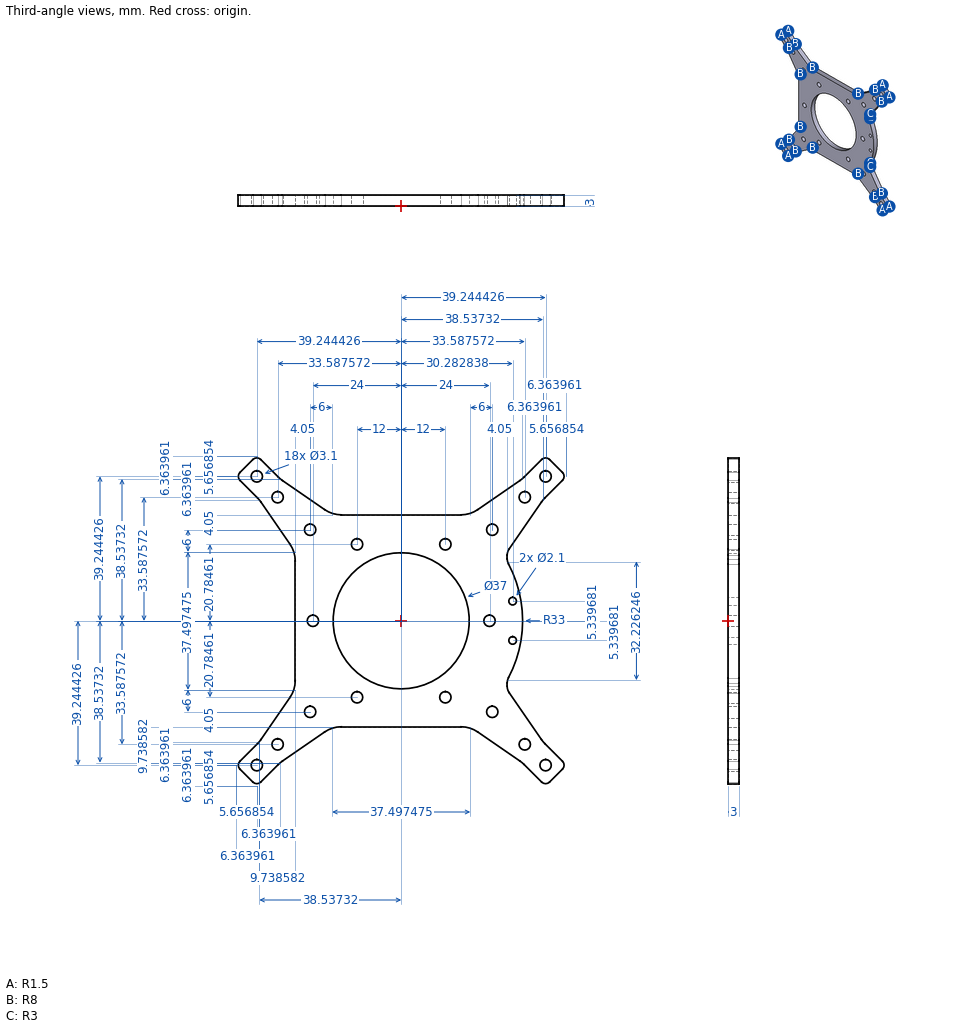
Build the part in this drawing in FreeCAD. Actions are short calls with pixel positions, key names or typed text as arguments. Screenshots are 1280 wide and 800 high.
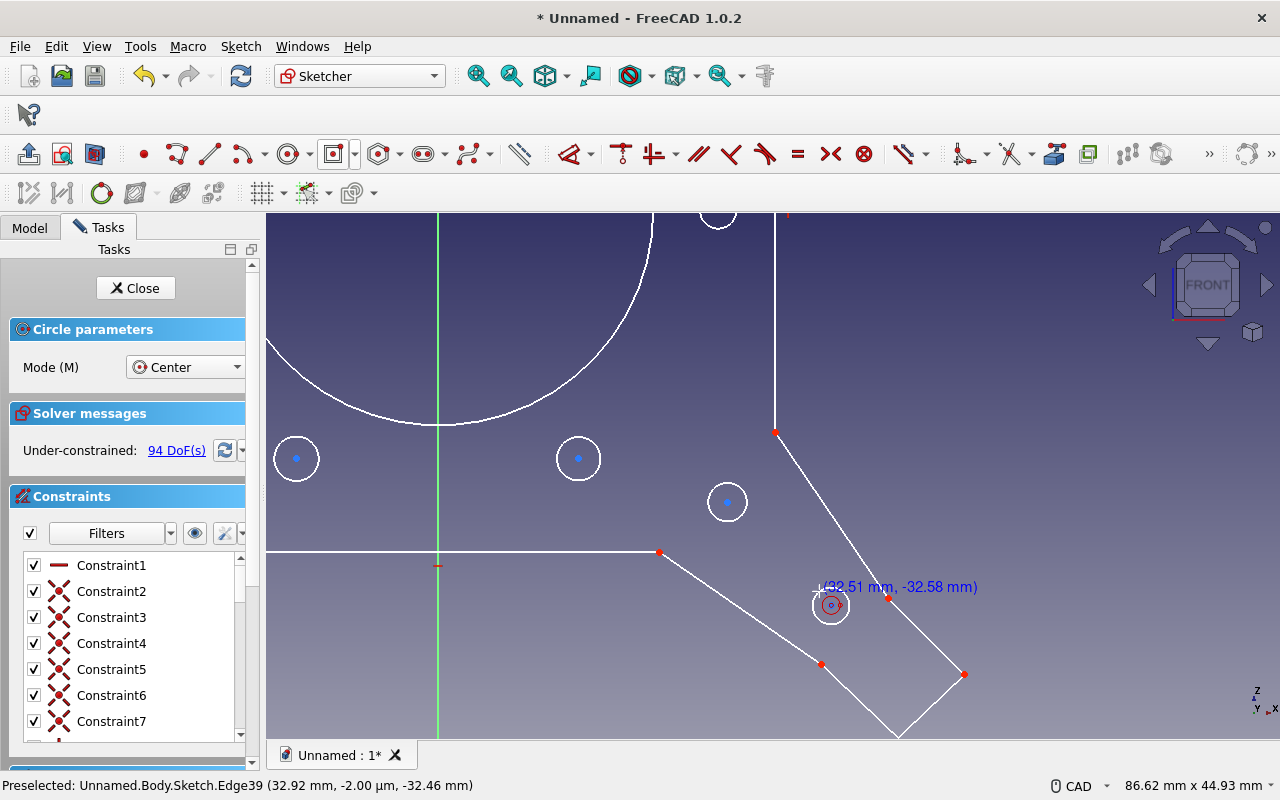
scroll(898, 670, up, 2)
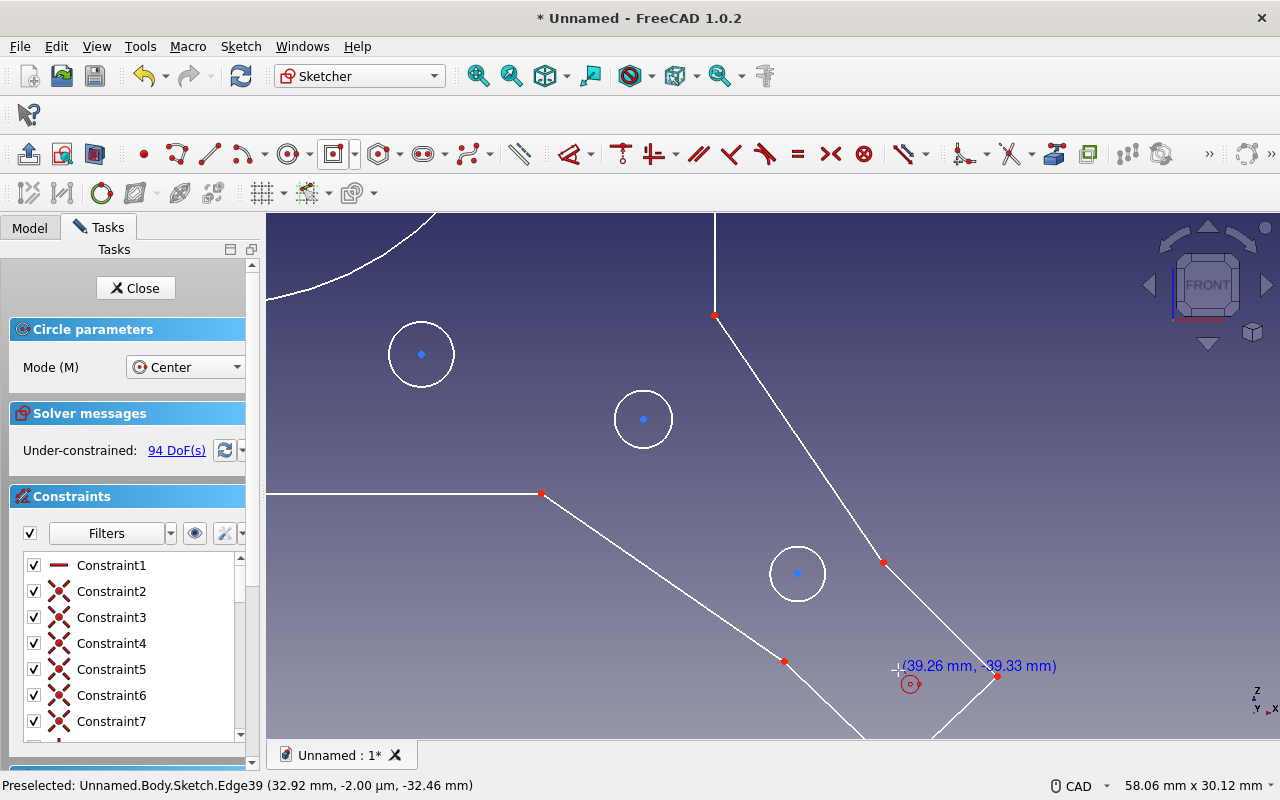
scroll(829, 600, down, 8)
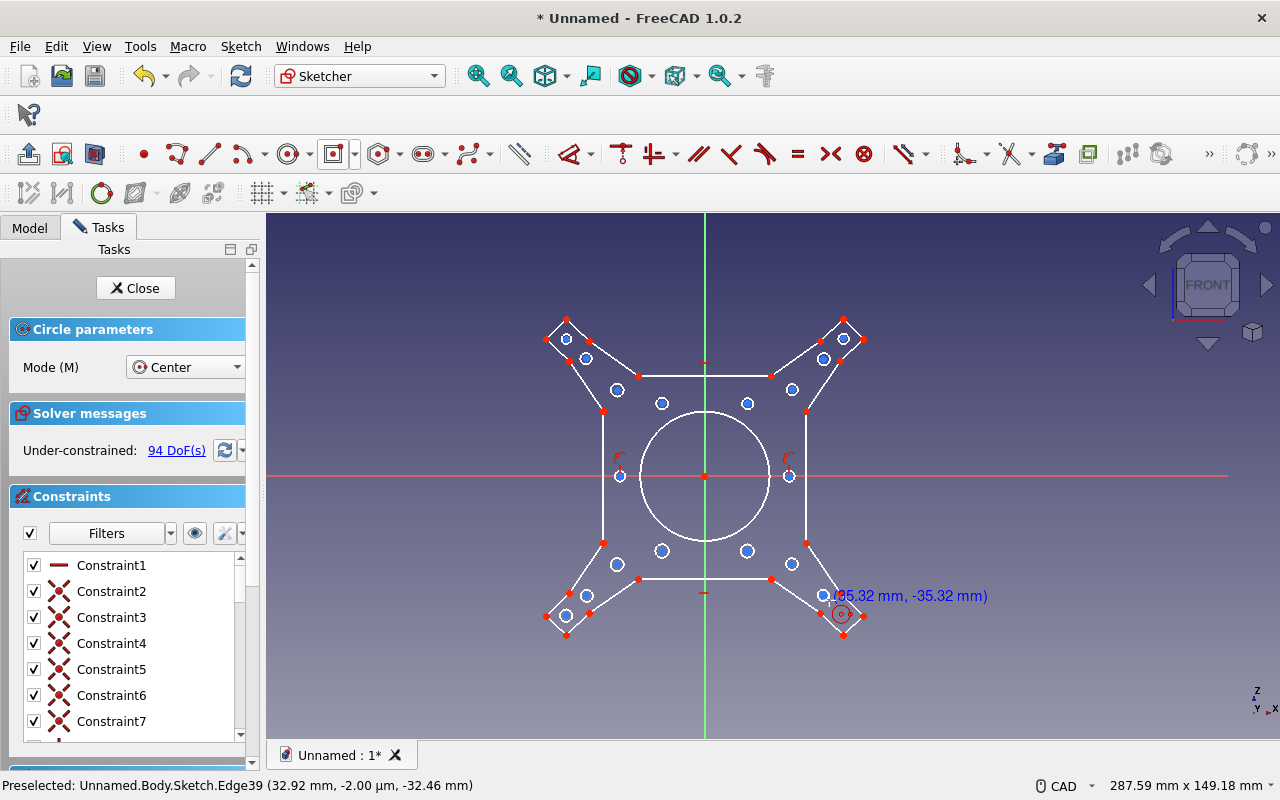
click(843, 615)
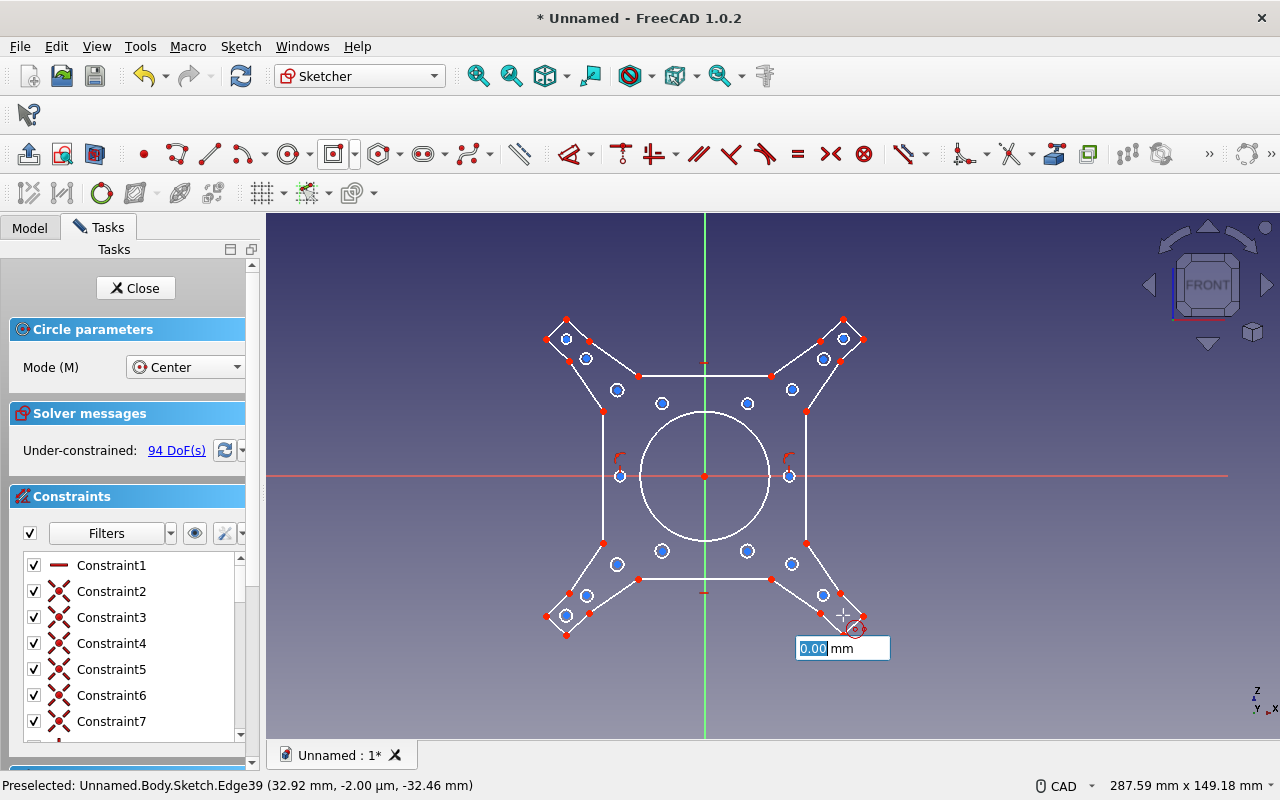
scroll(839, 611, up, 6)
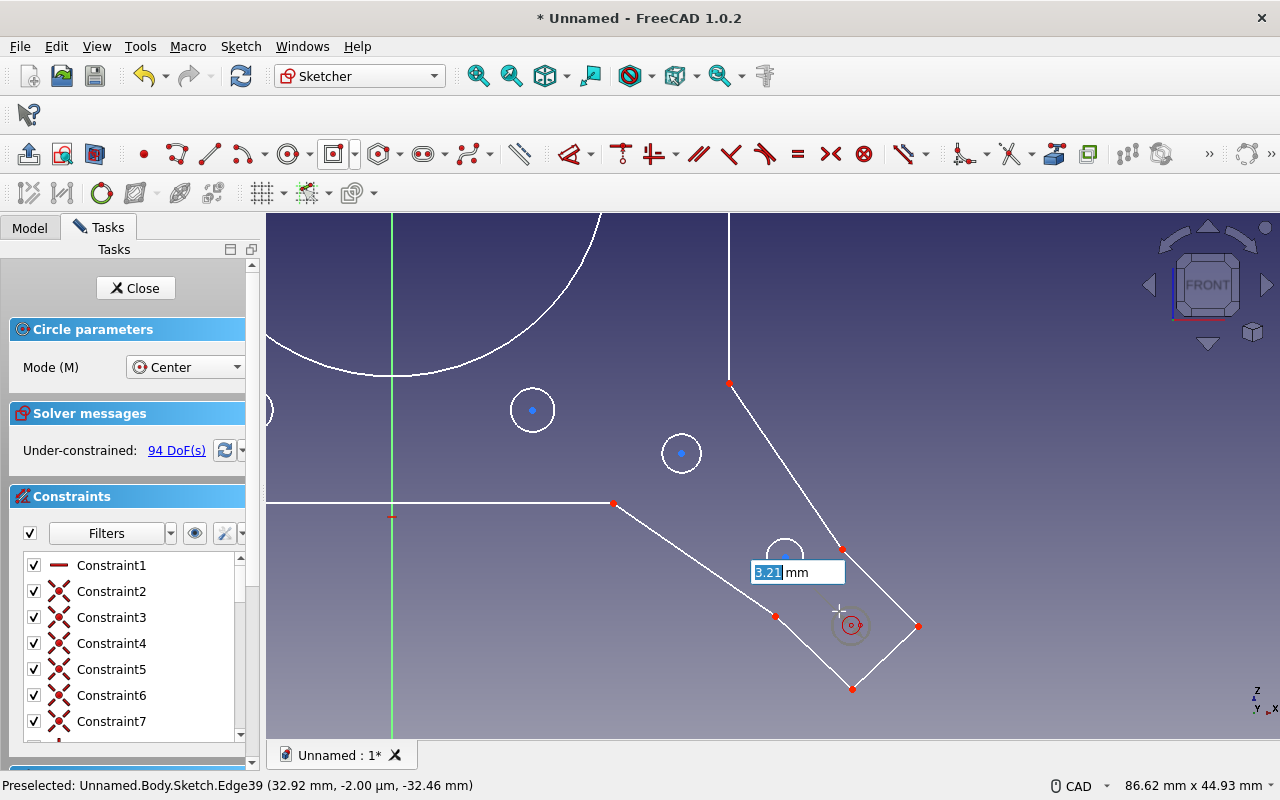
click(839, 608)
key(Escape)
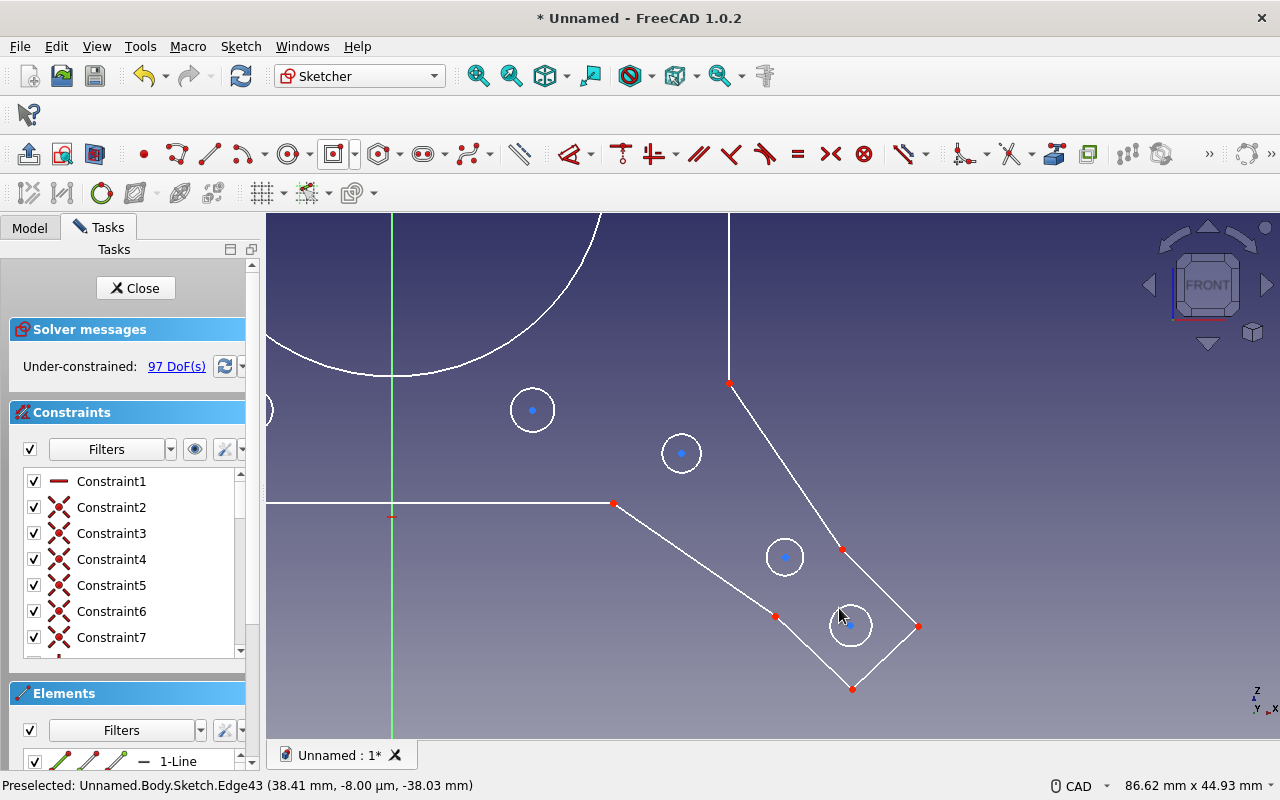
scroll(839, 611, down, 6)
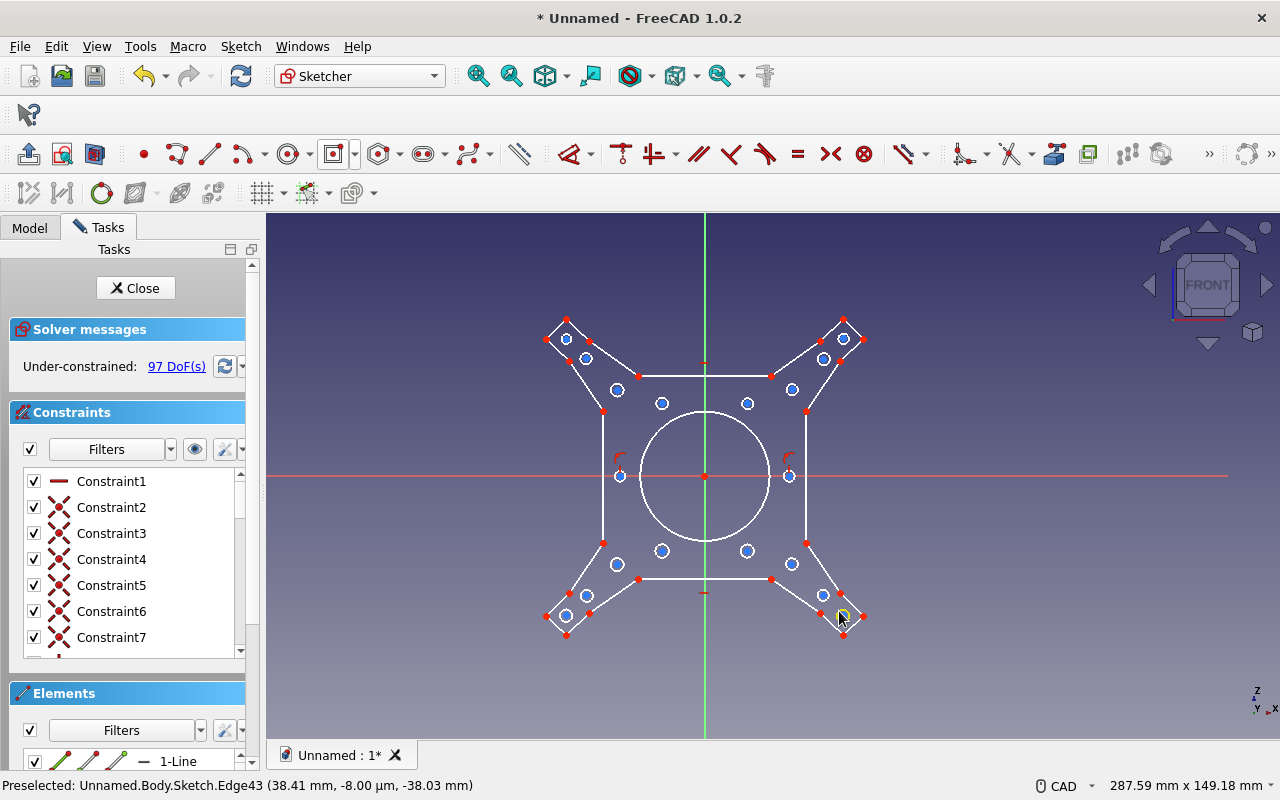
scroll(570, 336, up, 6)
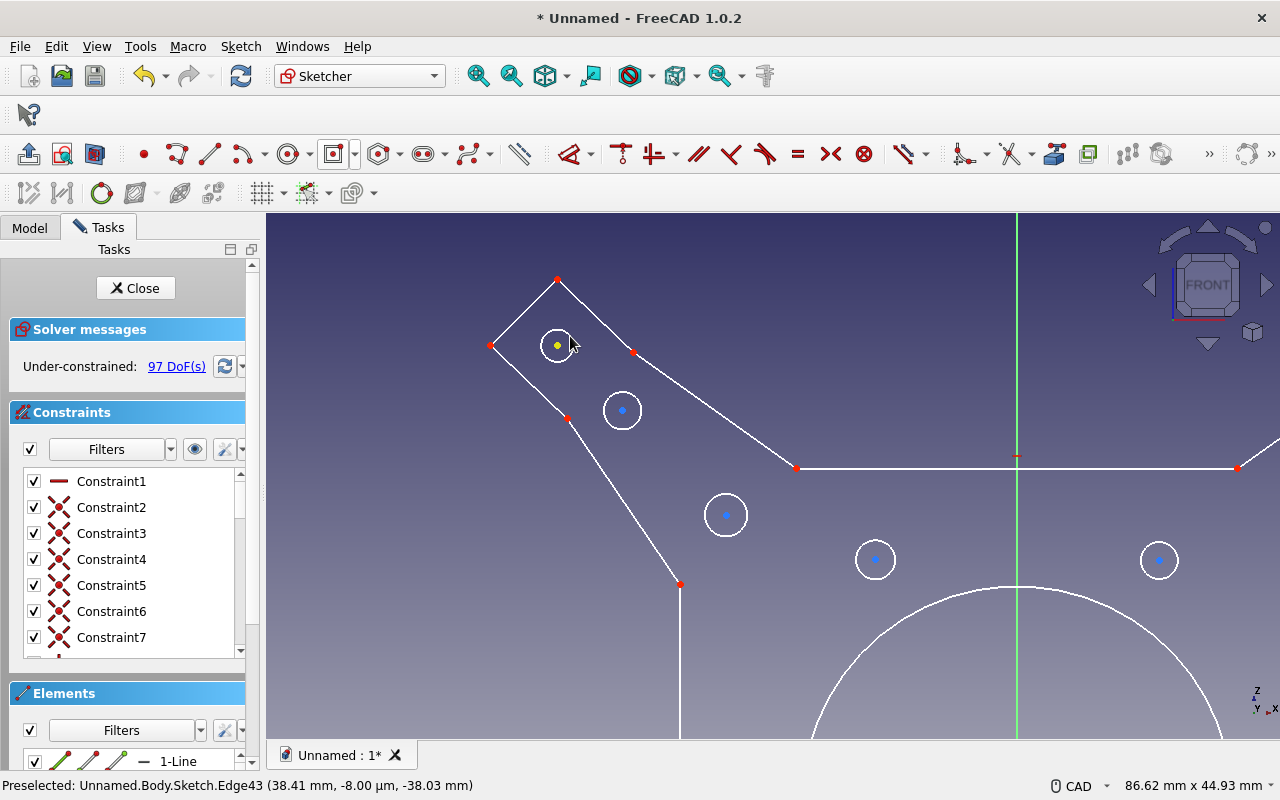
click(569, 334)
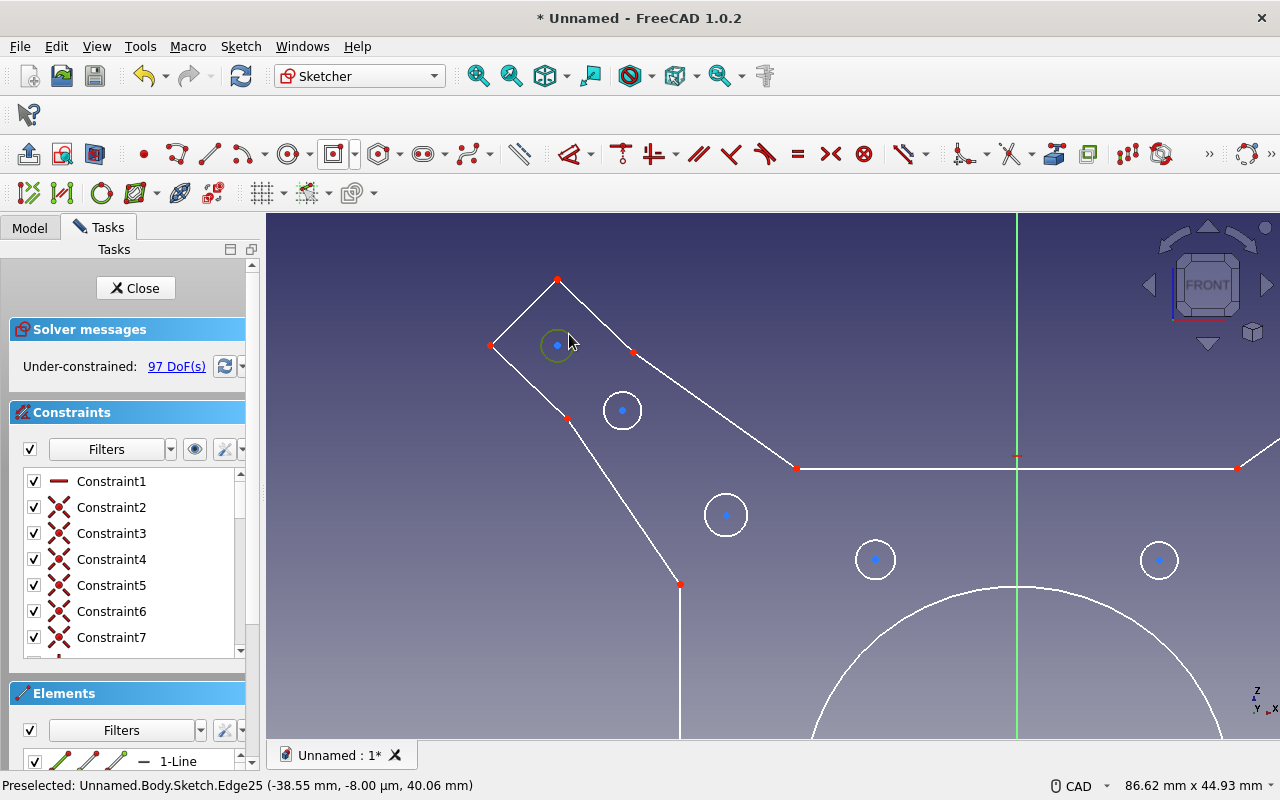
click(636, 397)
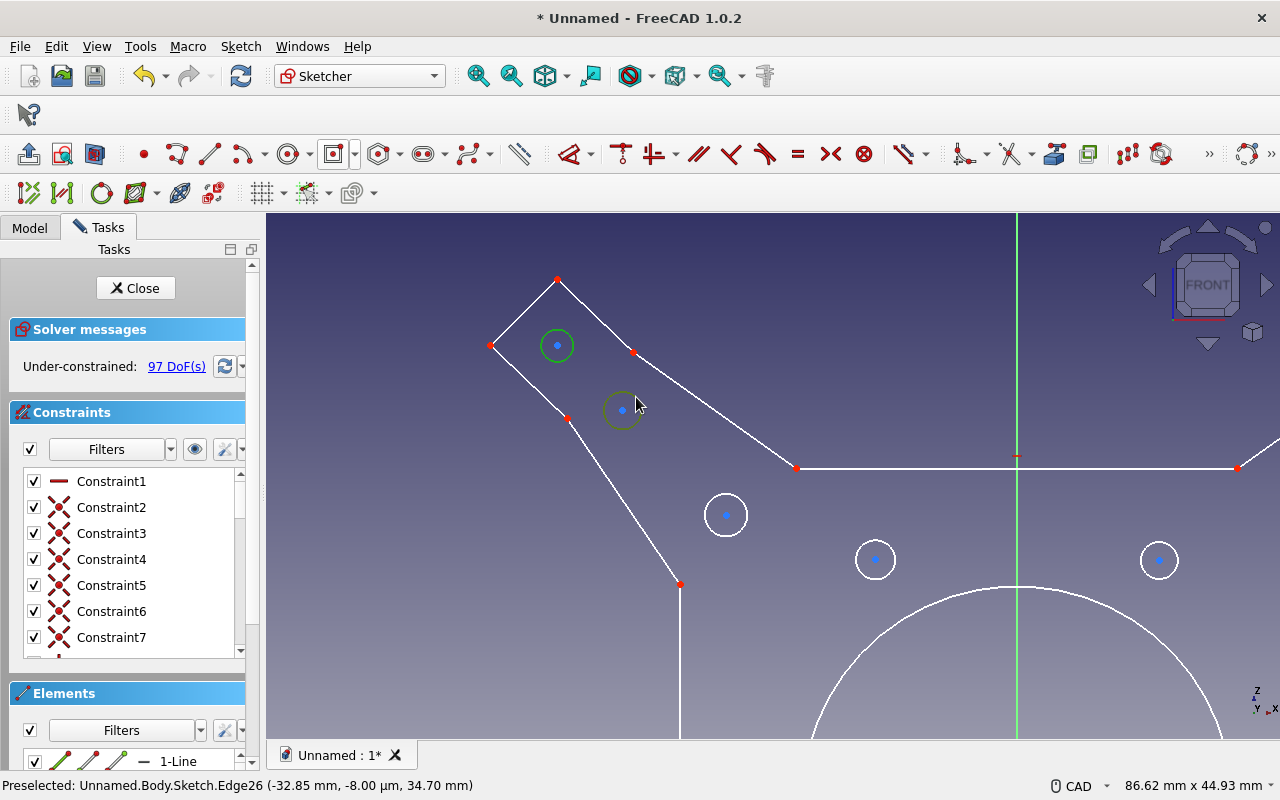
click(741, 500)